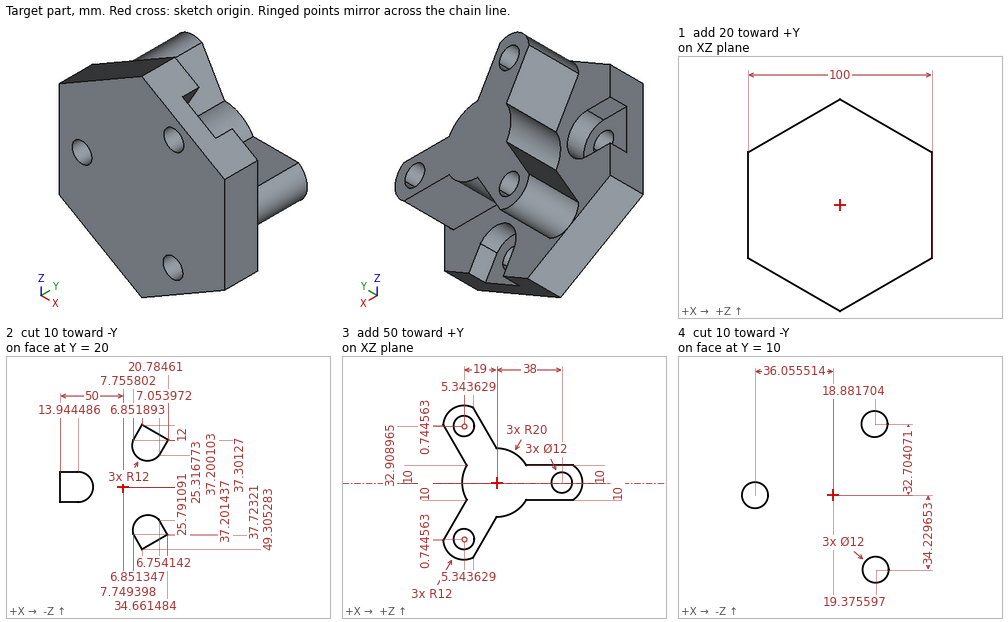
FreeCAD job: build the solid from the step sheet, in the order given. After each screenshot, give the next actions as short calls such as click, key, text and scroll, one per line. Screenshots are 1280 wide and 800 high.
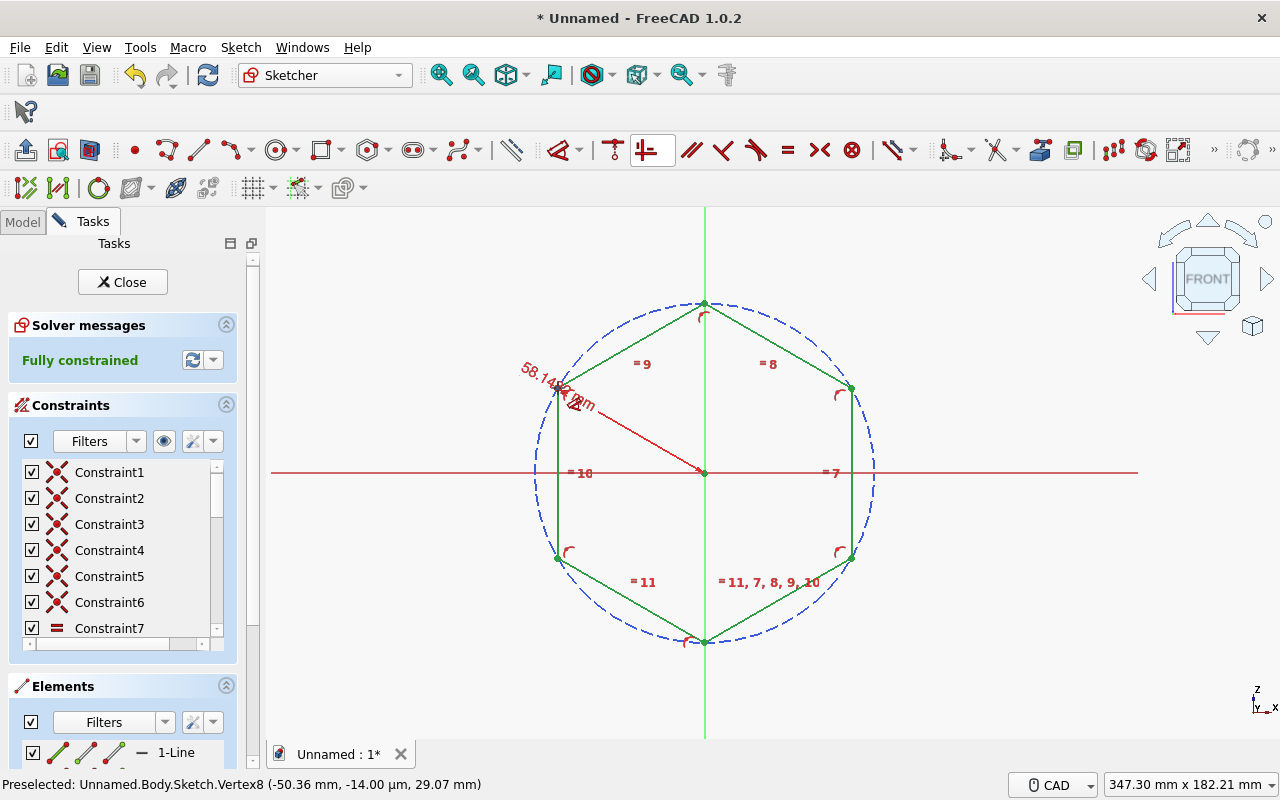
click(852, 558)
click(602, 640)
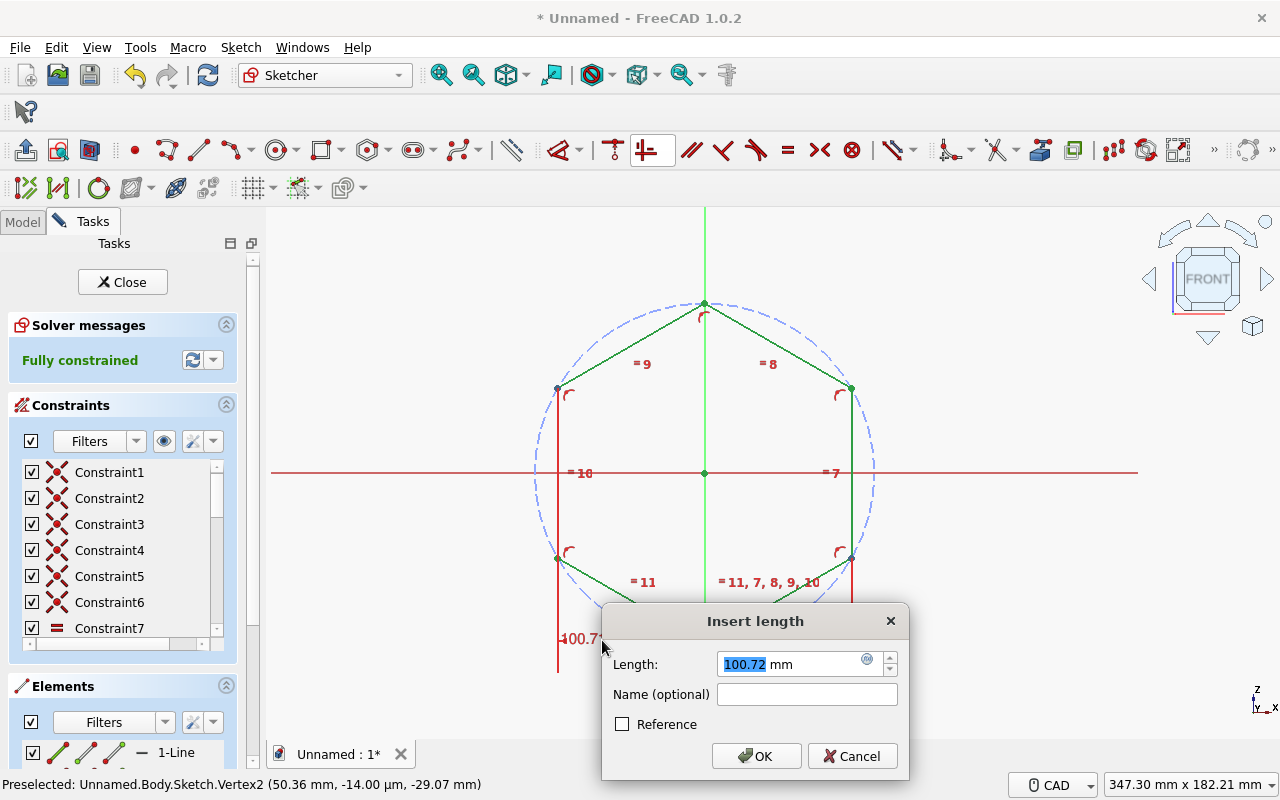
text(100)
key(Return)
key(Escape)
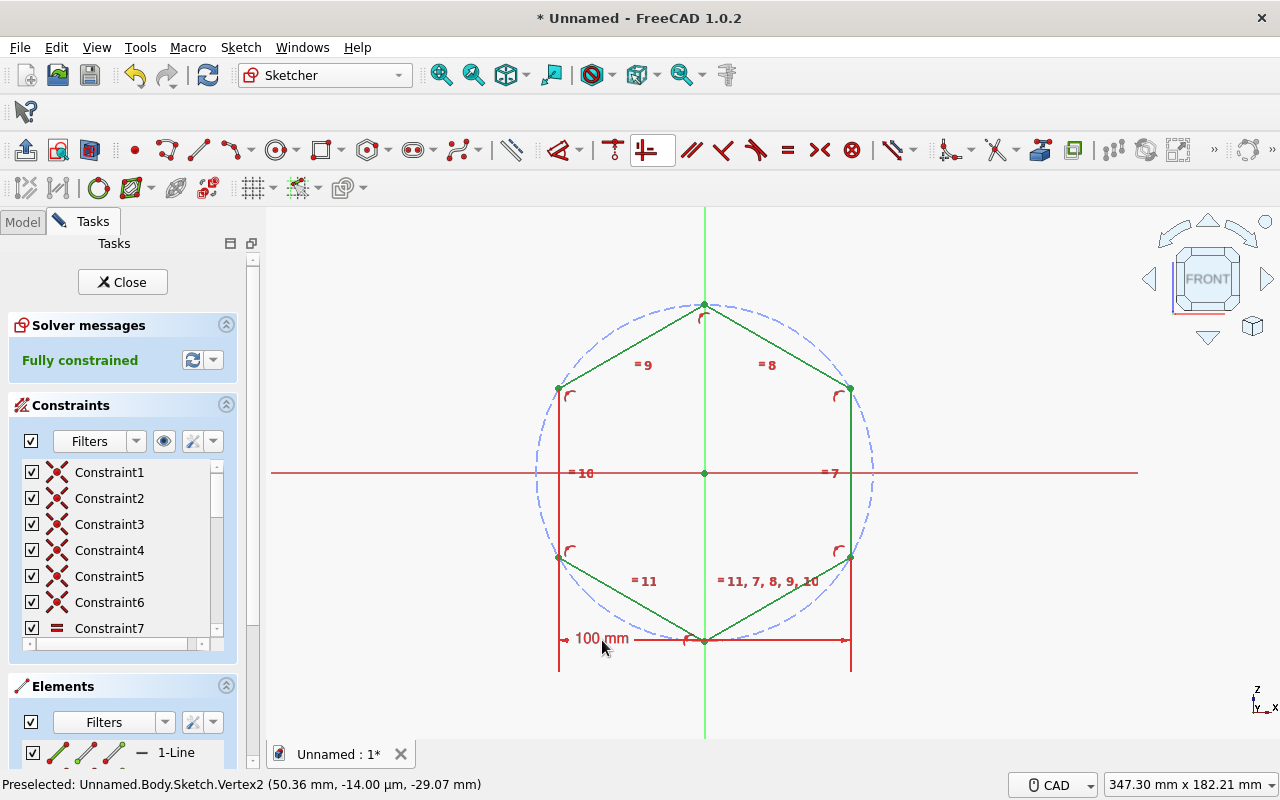
click(123, 282)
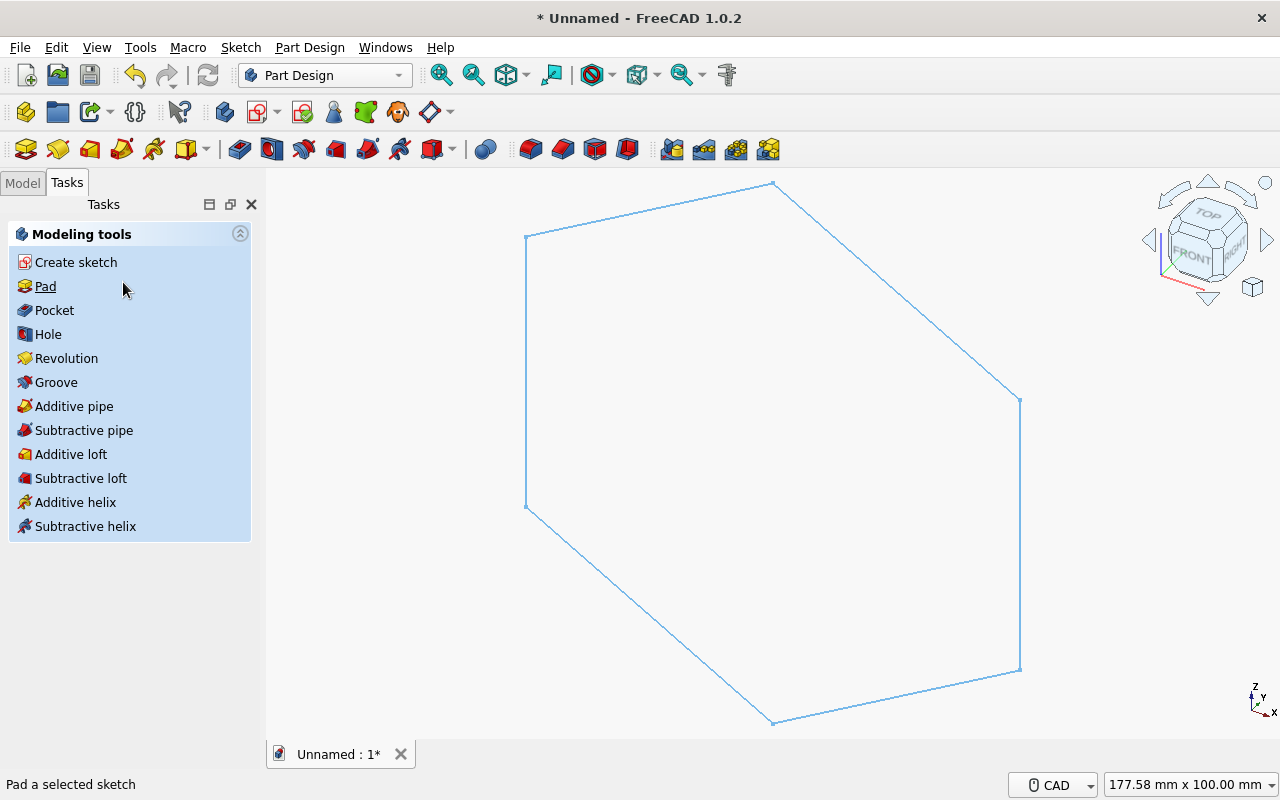
click(26, 150)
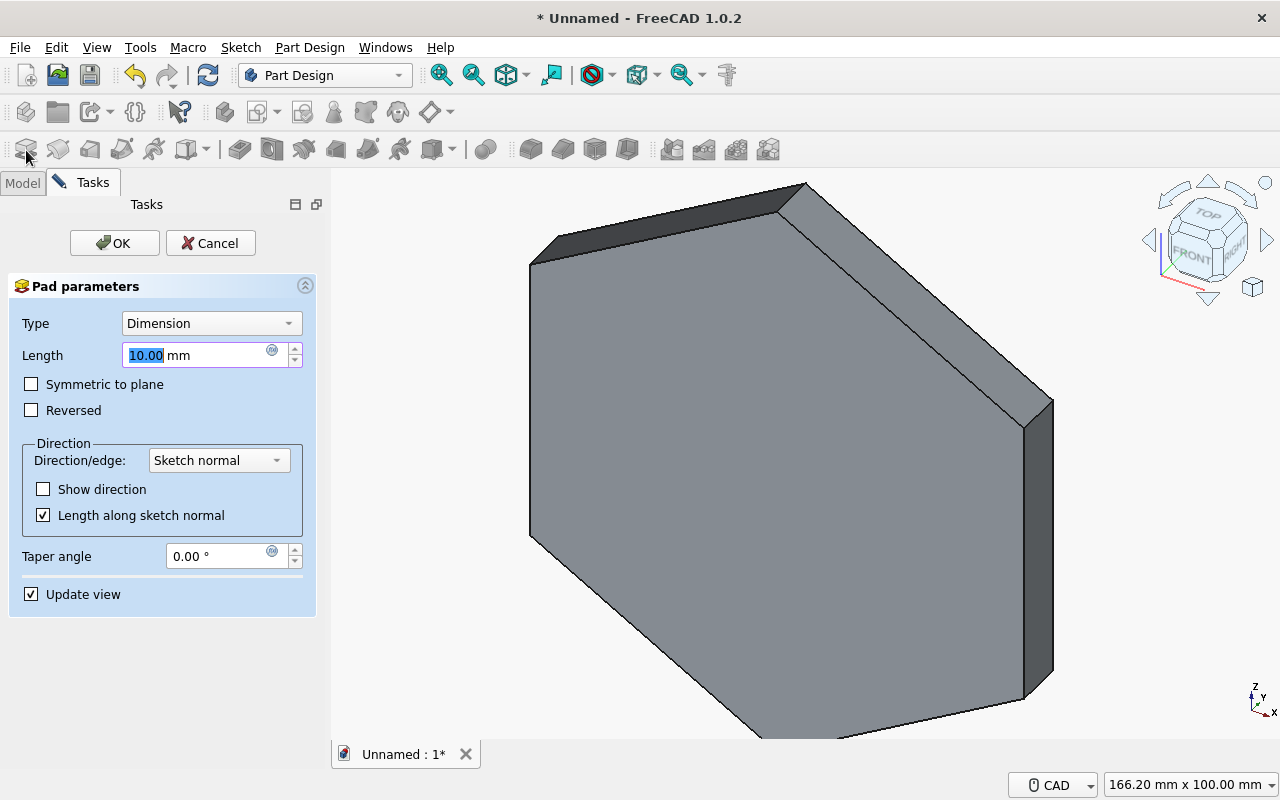
text(20)
key(Tab)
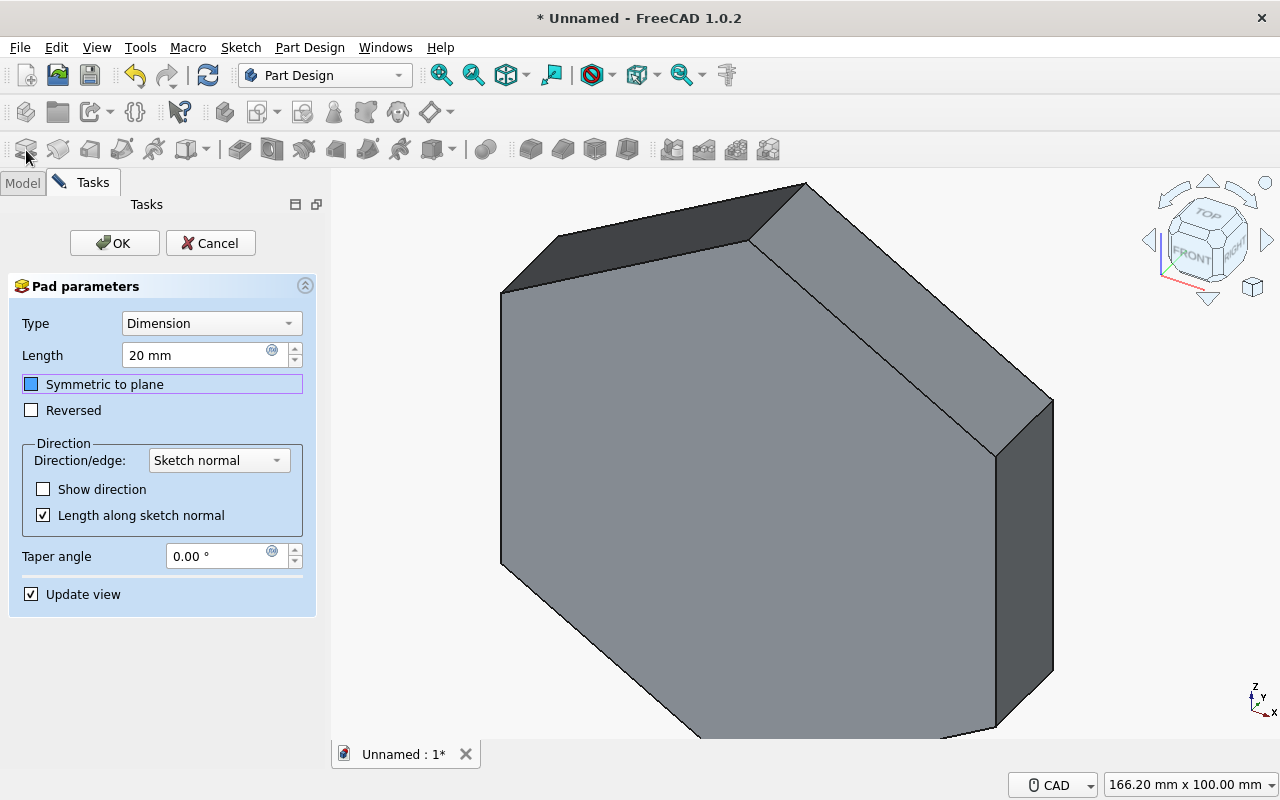
click(30, 410)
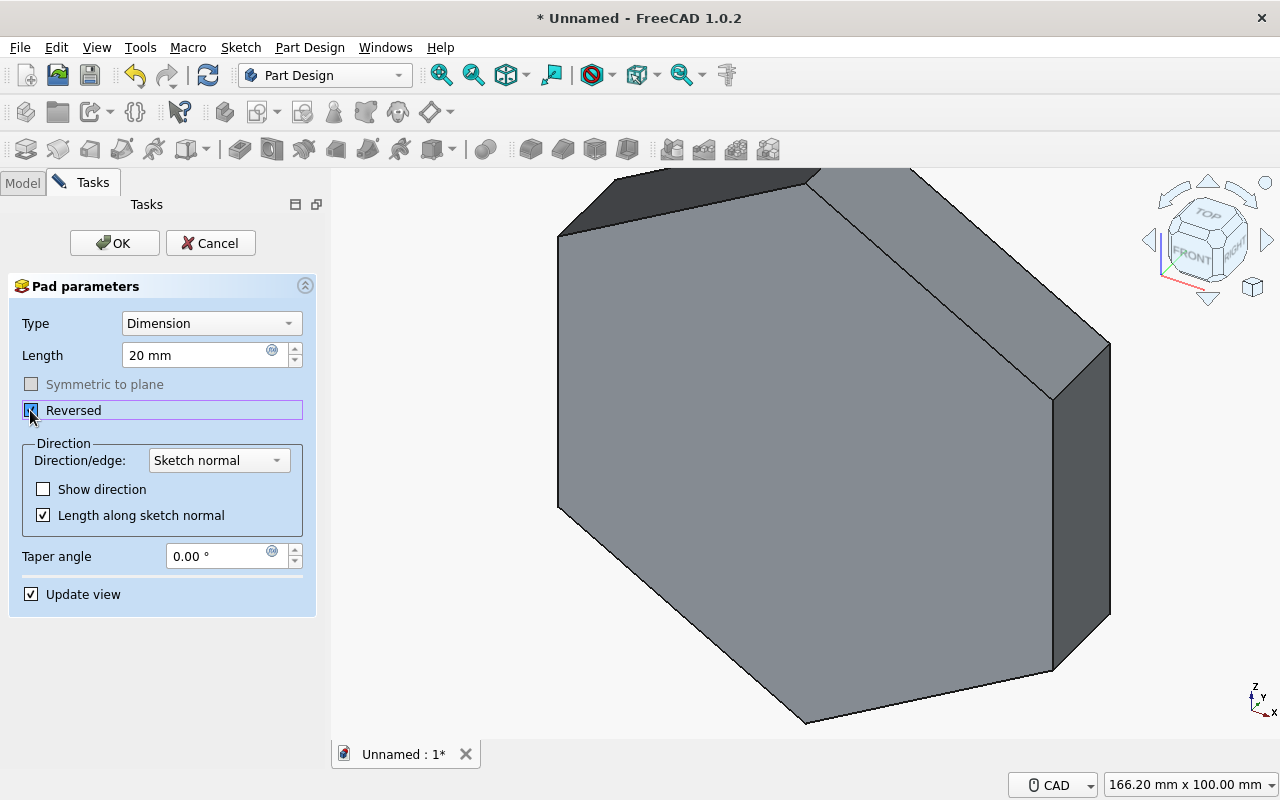
click(115, 243)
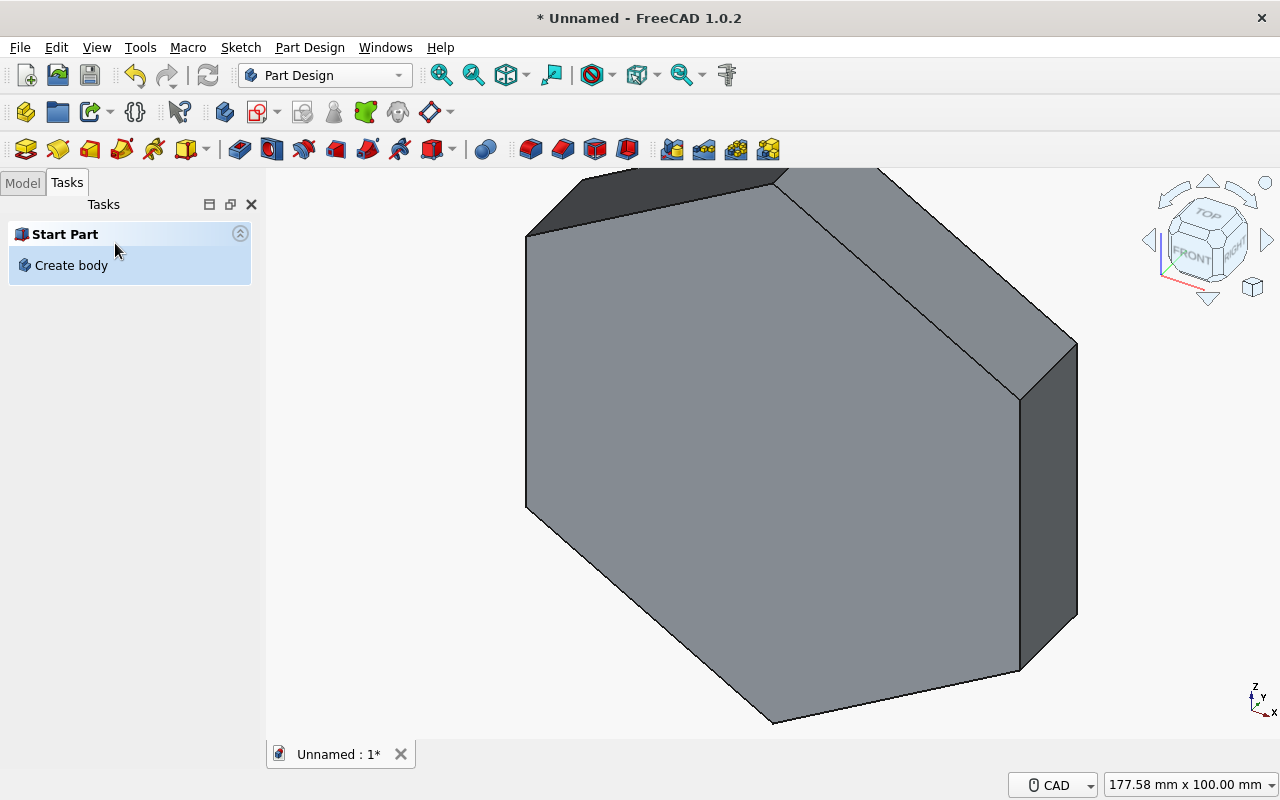
key(v)
key(f)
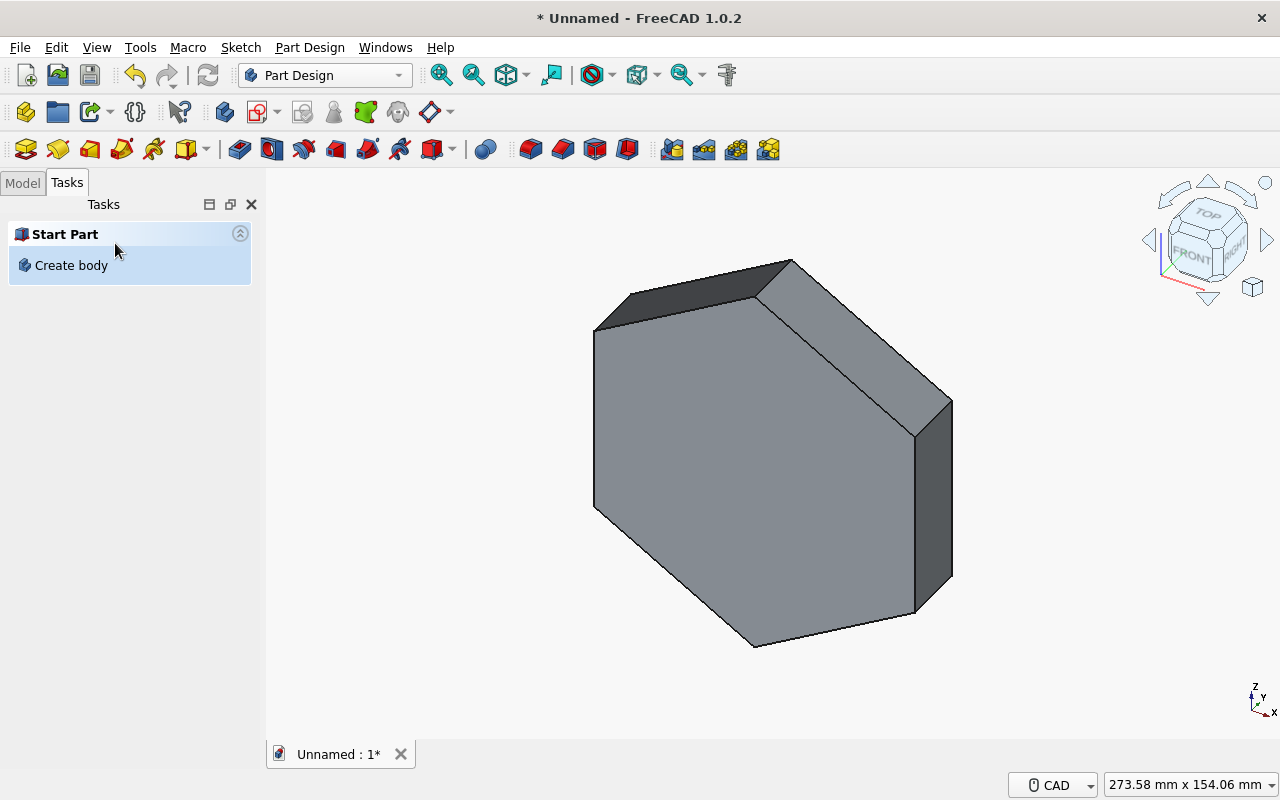
key(4)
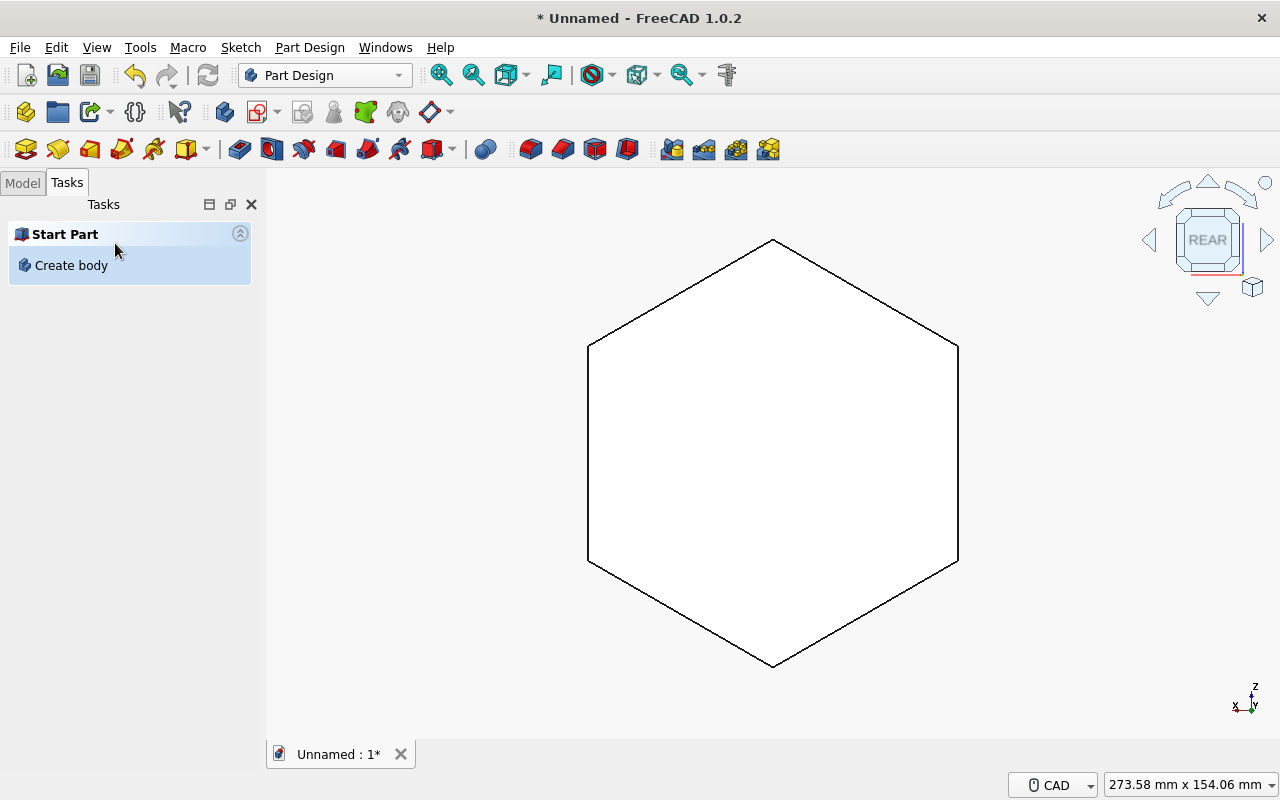
click(773, 453)